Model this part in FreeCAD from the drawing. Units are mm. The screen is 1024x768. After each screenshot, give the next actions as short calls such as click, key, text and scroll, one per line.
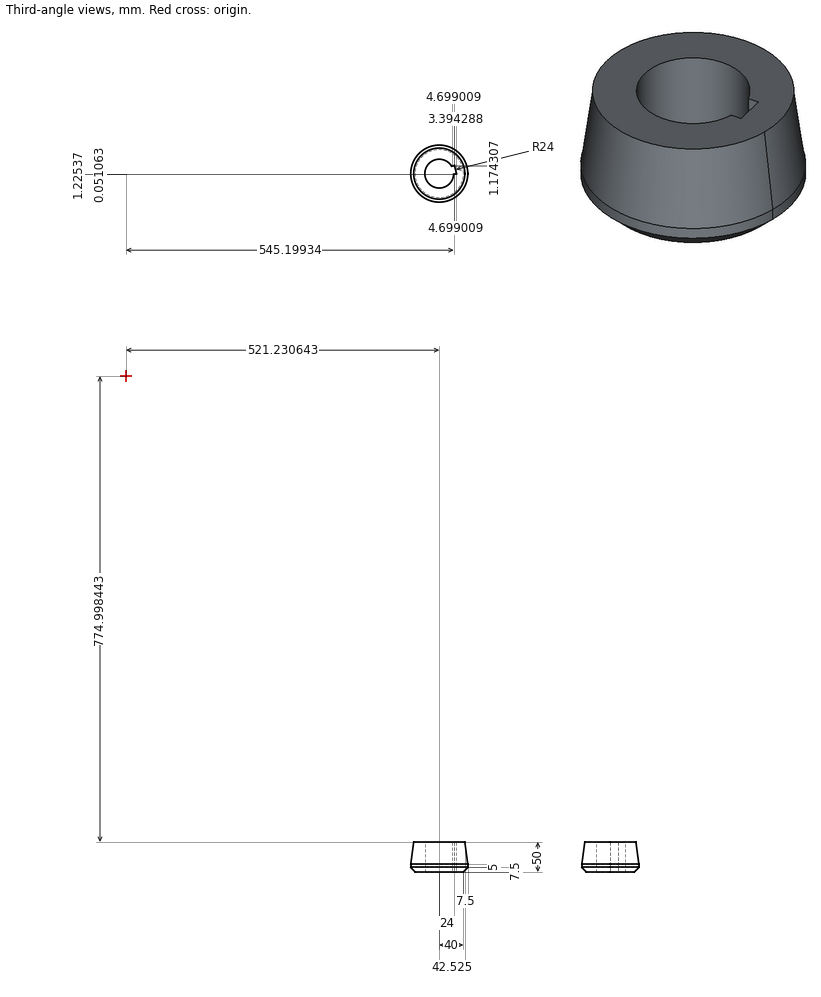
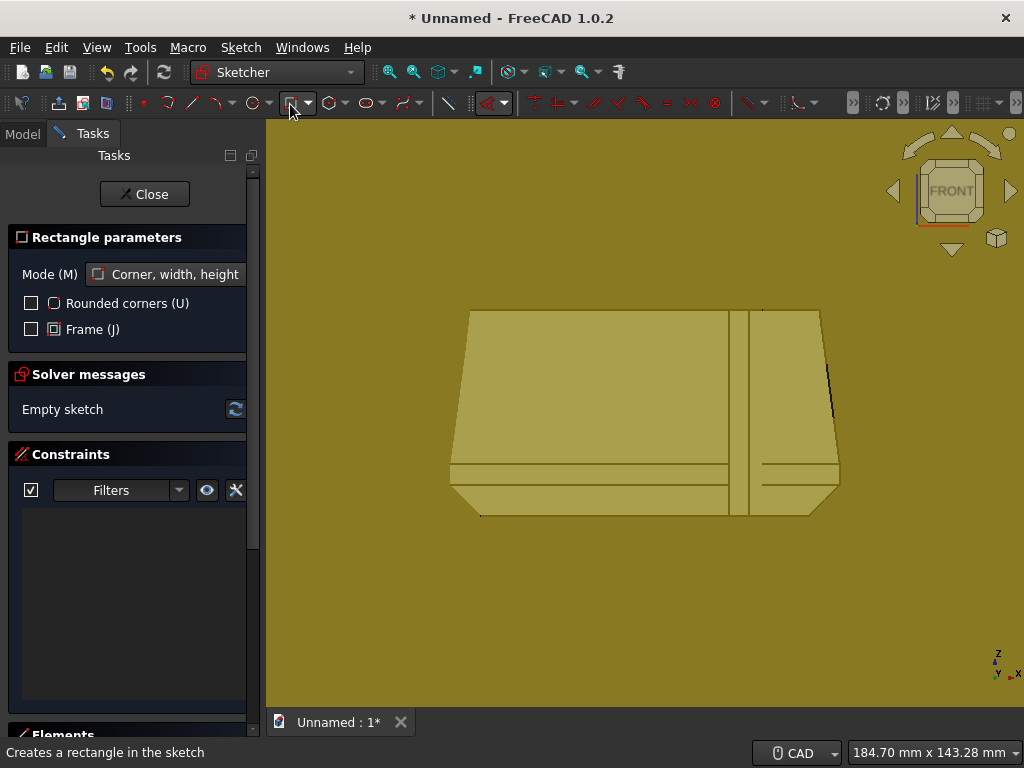
click(645, 310)
click(743, 516)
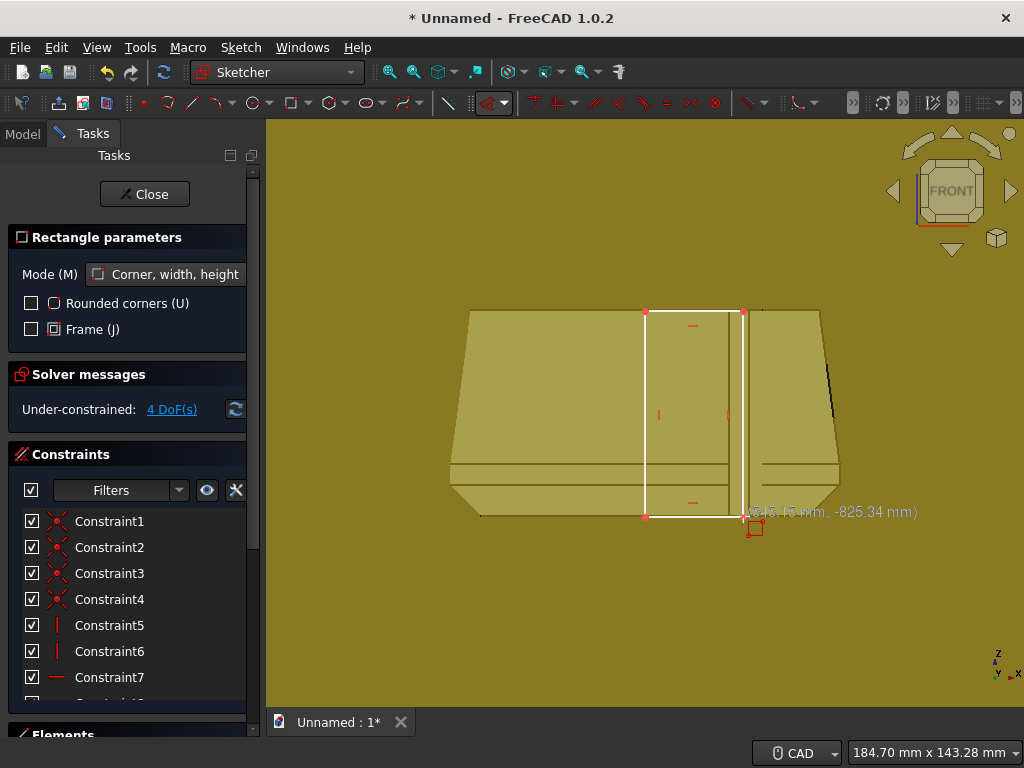
click(192, 104)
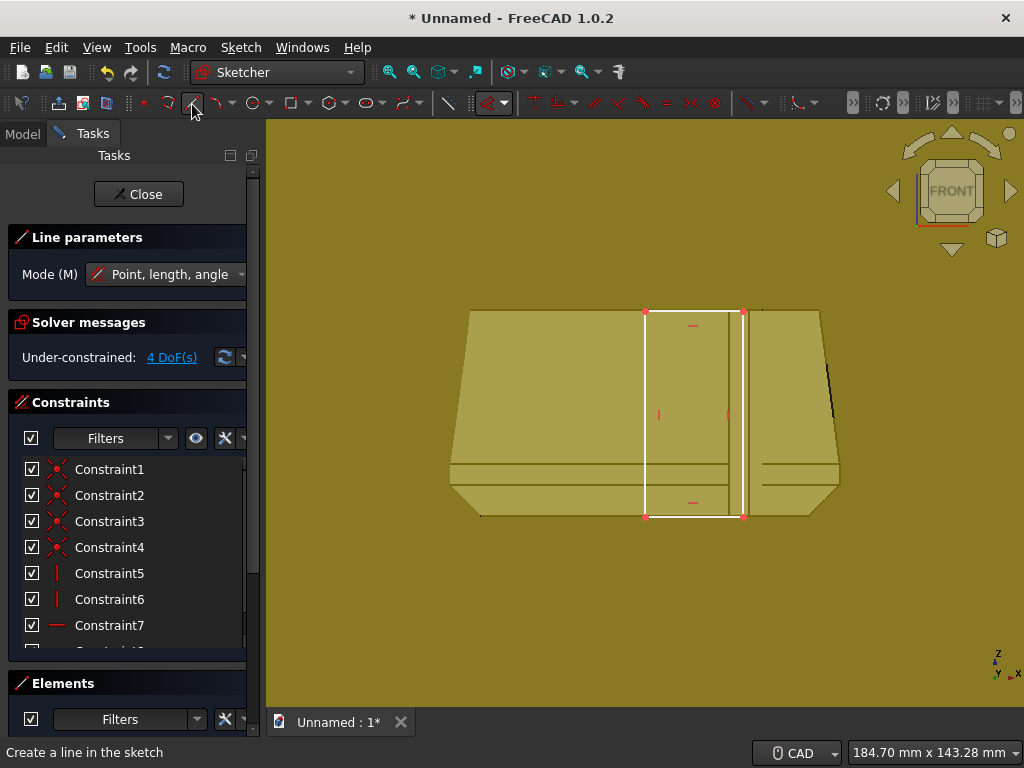
click(645, 536)
click(645, 598)
key(Escape)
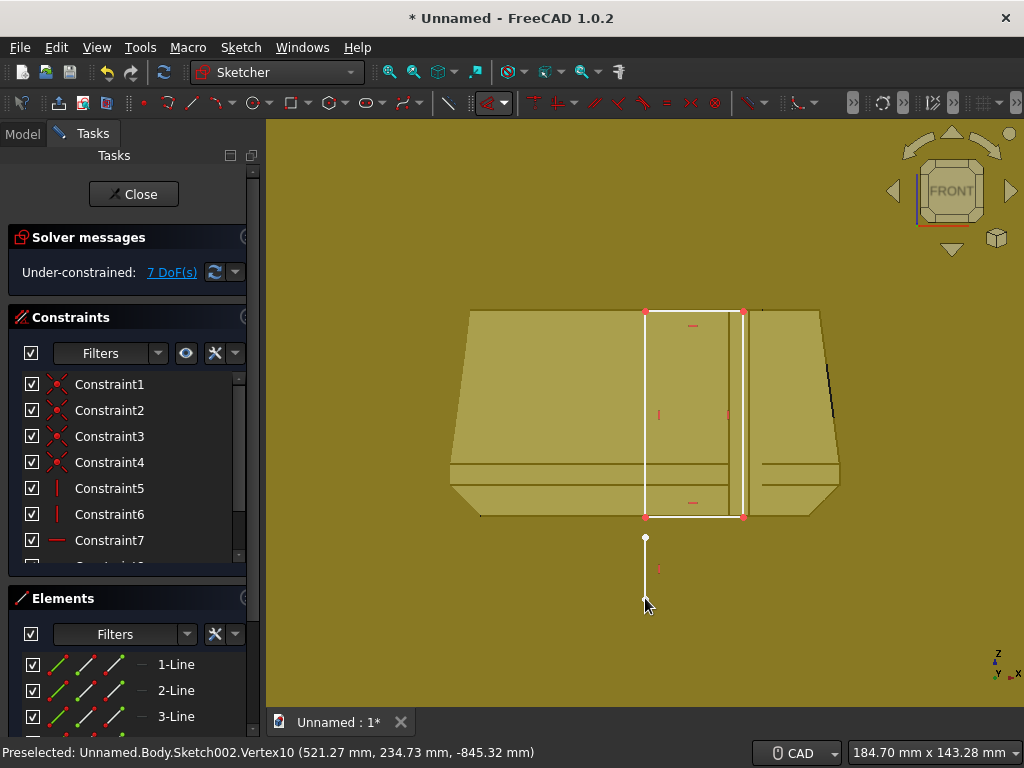
click(645, 556)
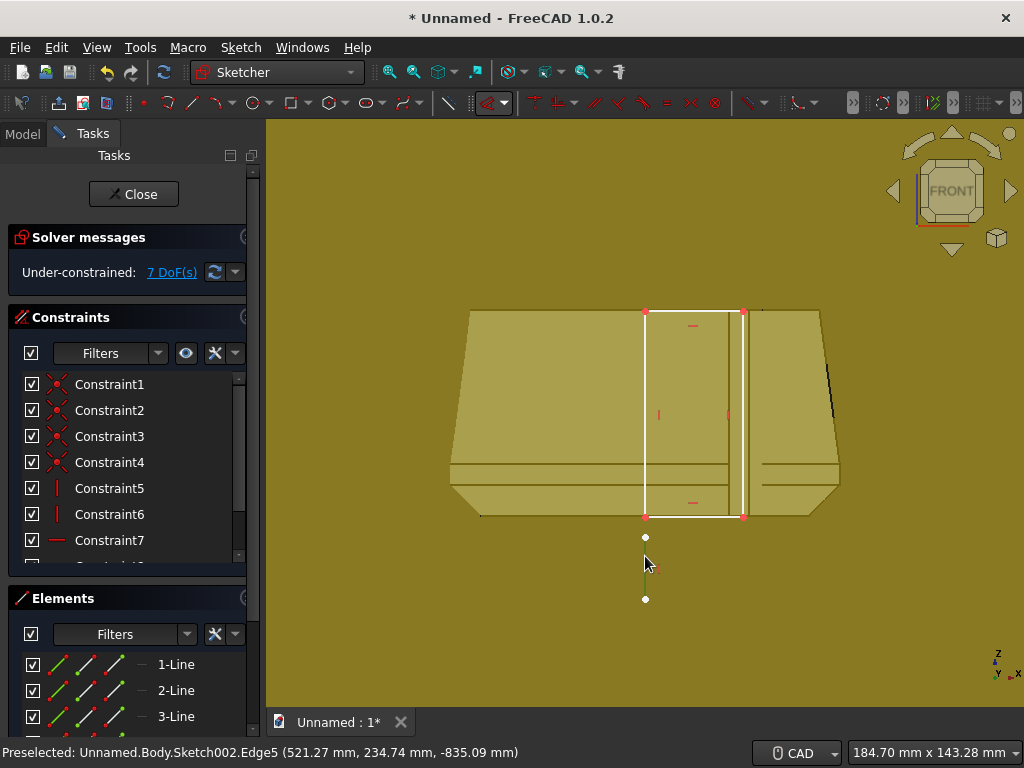
click(450, 104)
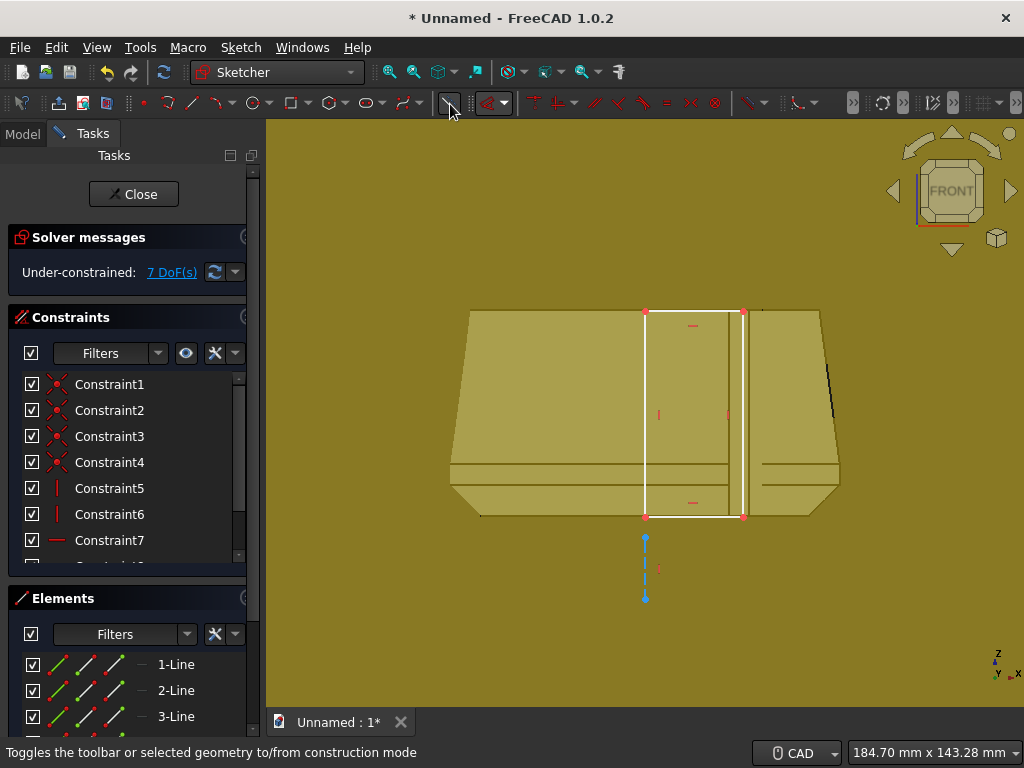
click(645, 373)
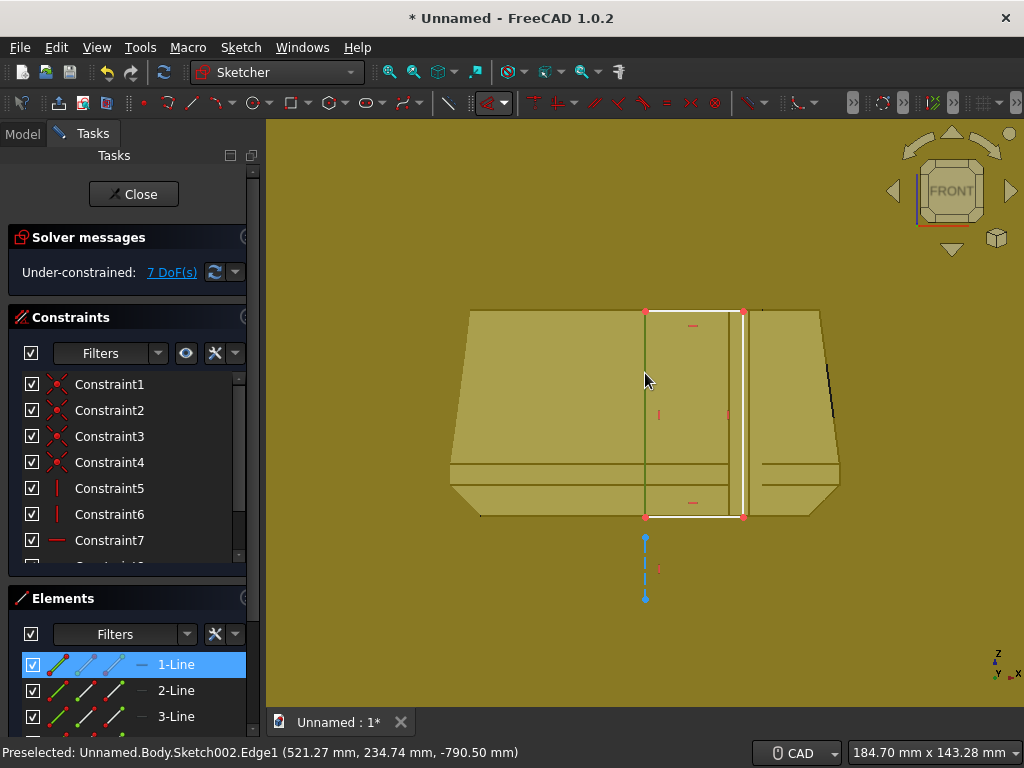
click(506, 104)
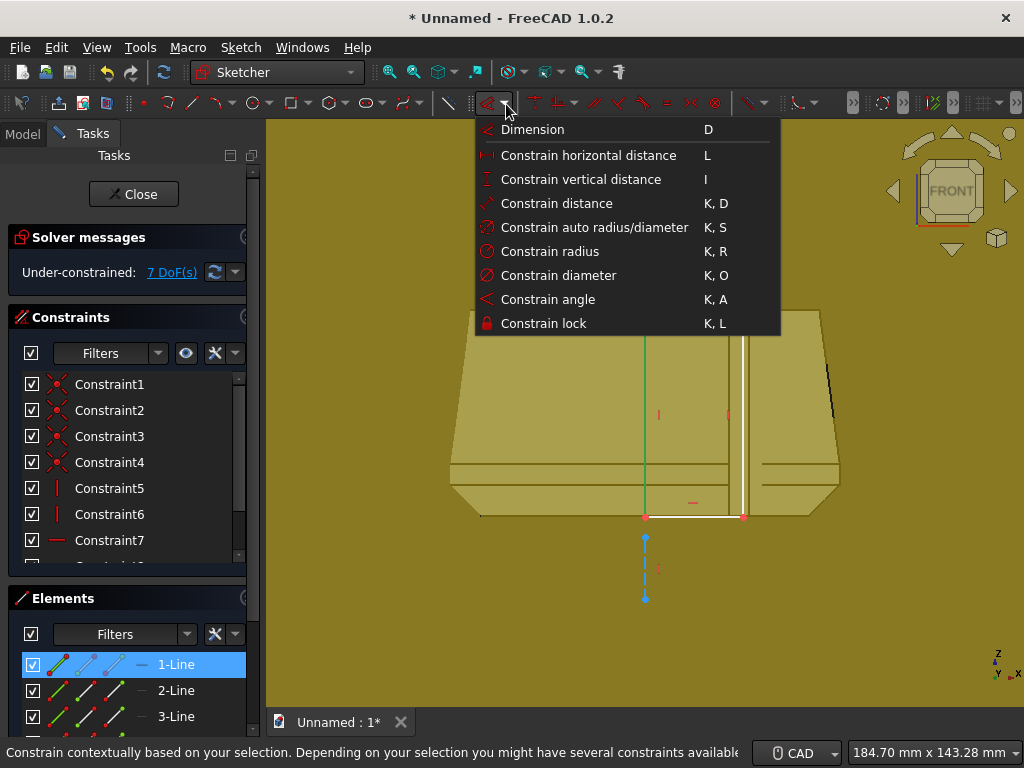
click(628, 179)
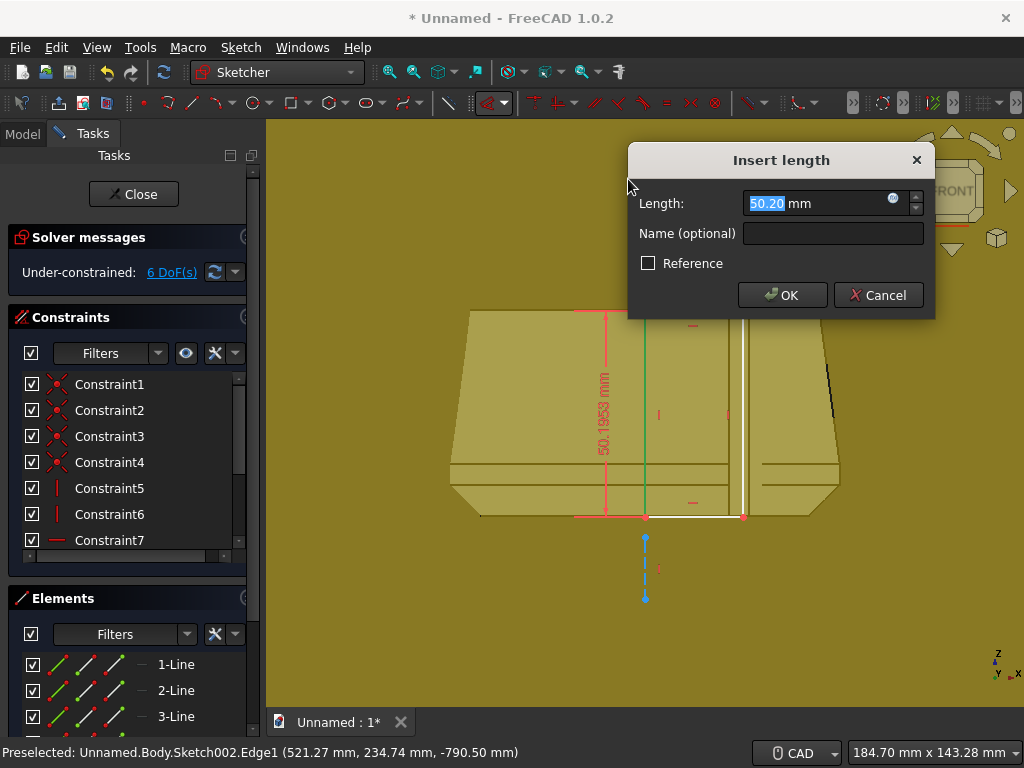
text(50)
key(Return)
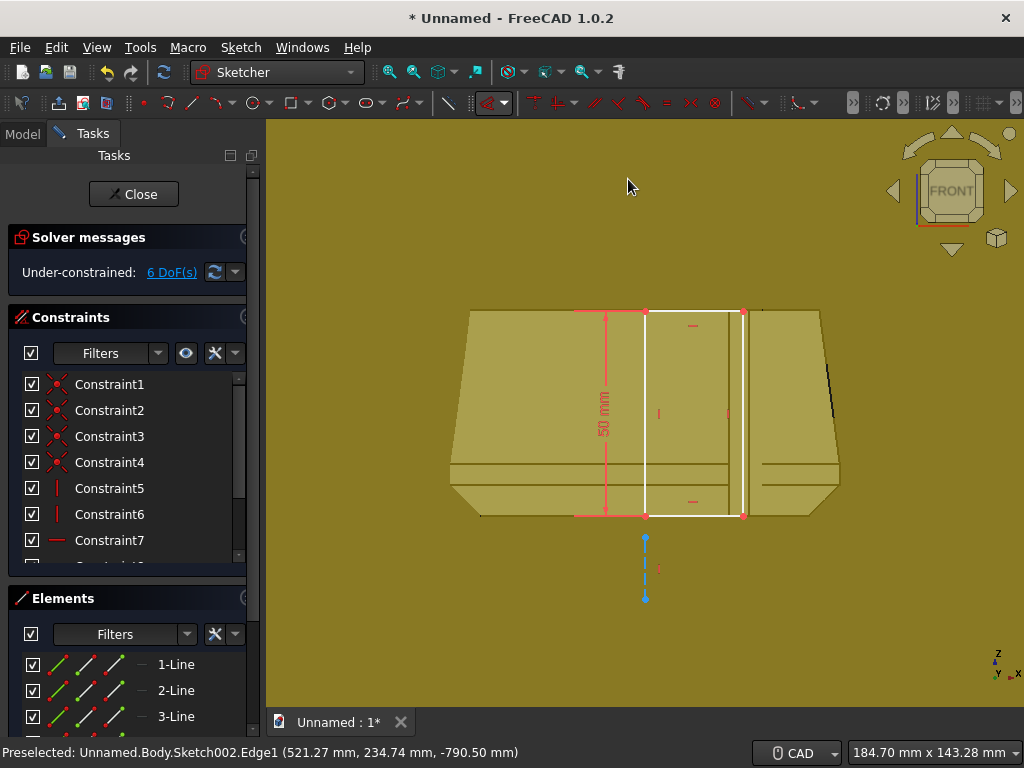
click(674, 516)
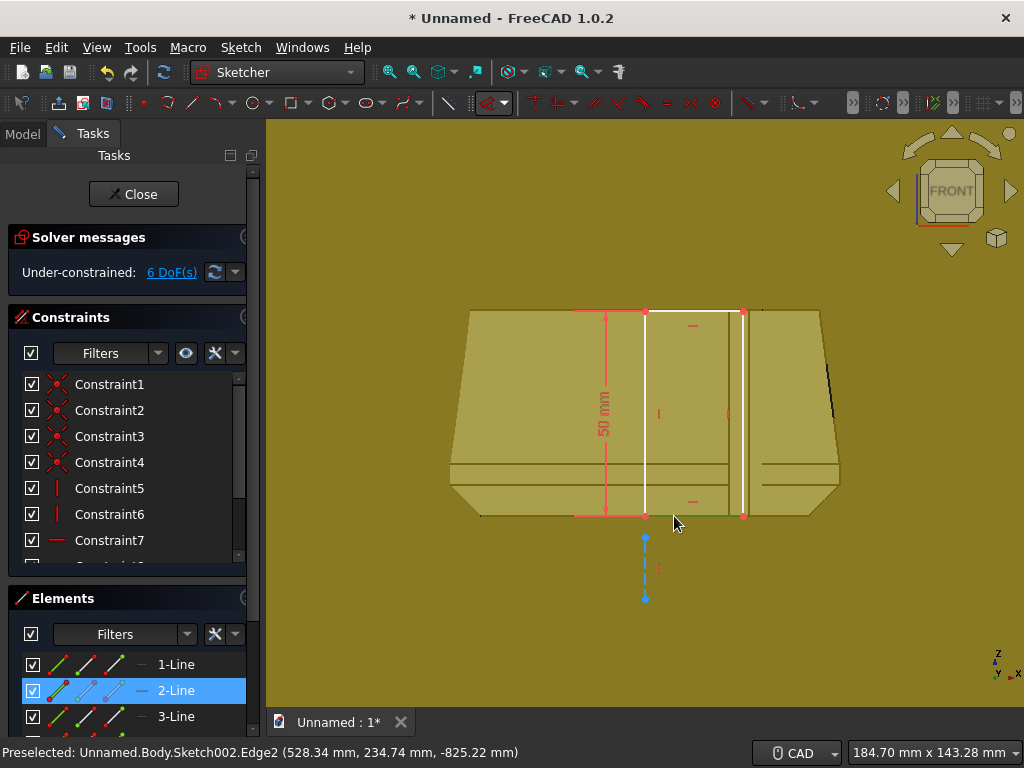
click(506, 104)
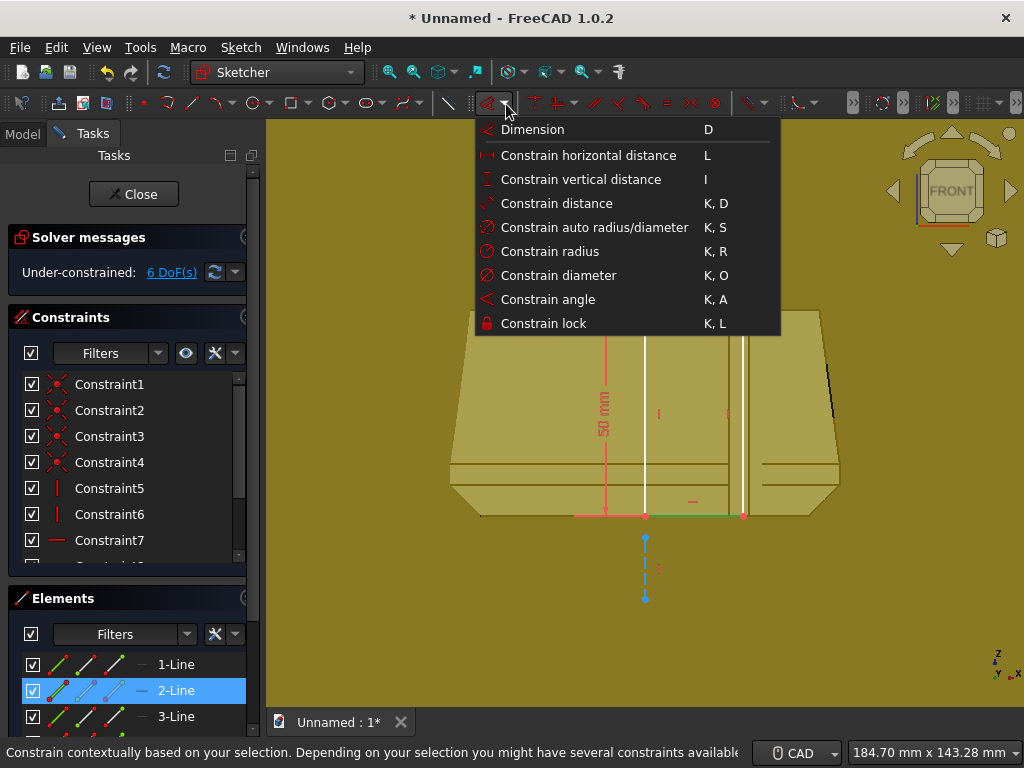
click(628, 155)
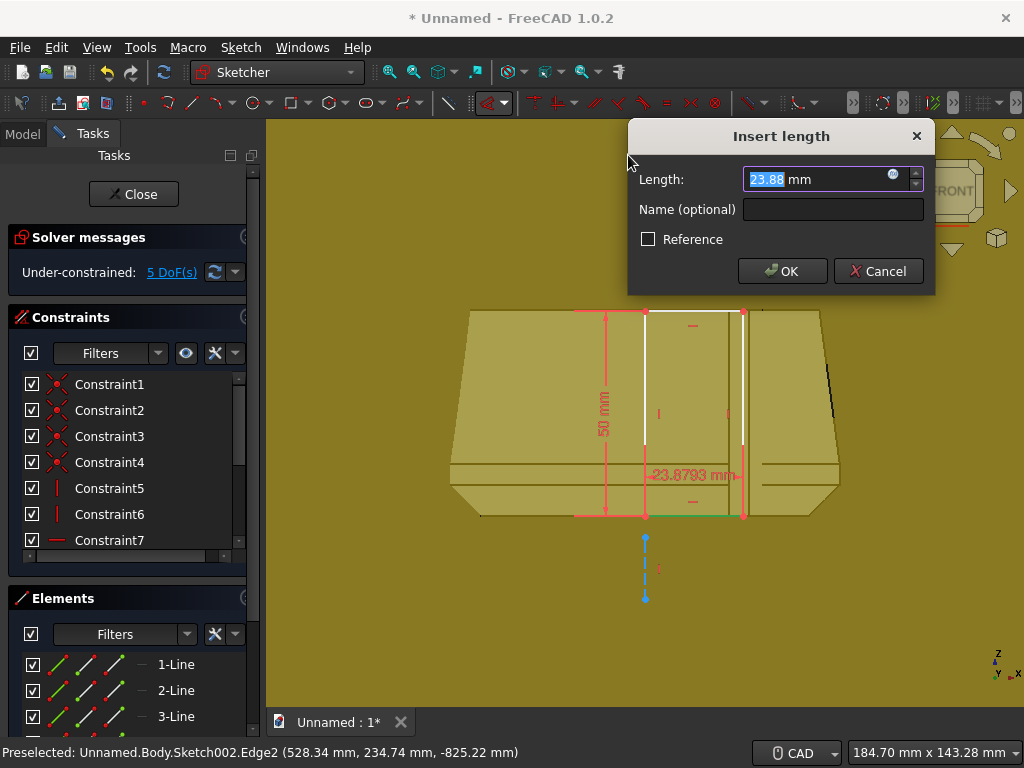
text(24)
key(Return)